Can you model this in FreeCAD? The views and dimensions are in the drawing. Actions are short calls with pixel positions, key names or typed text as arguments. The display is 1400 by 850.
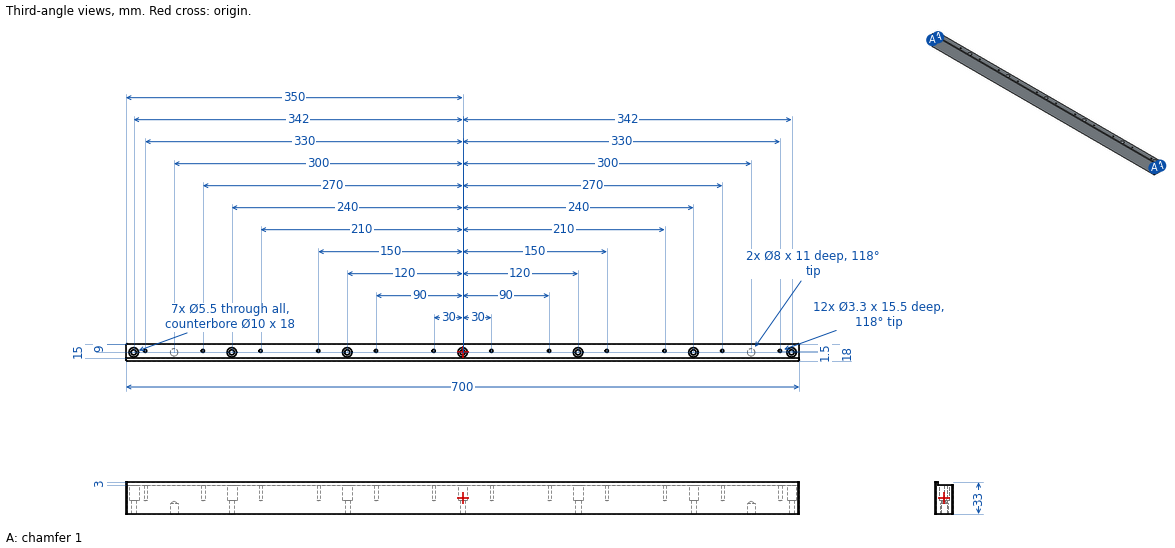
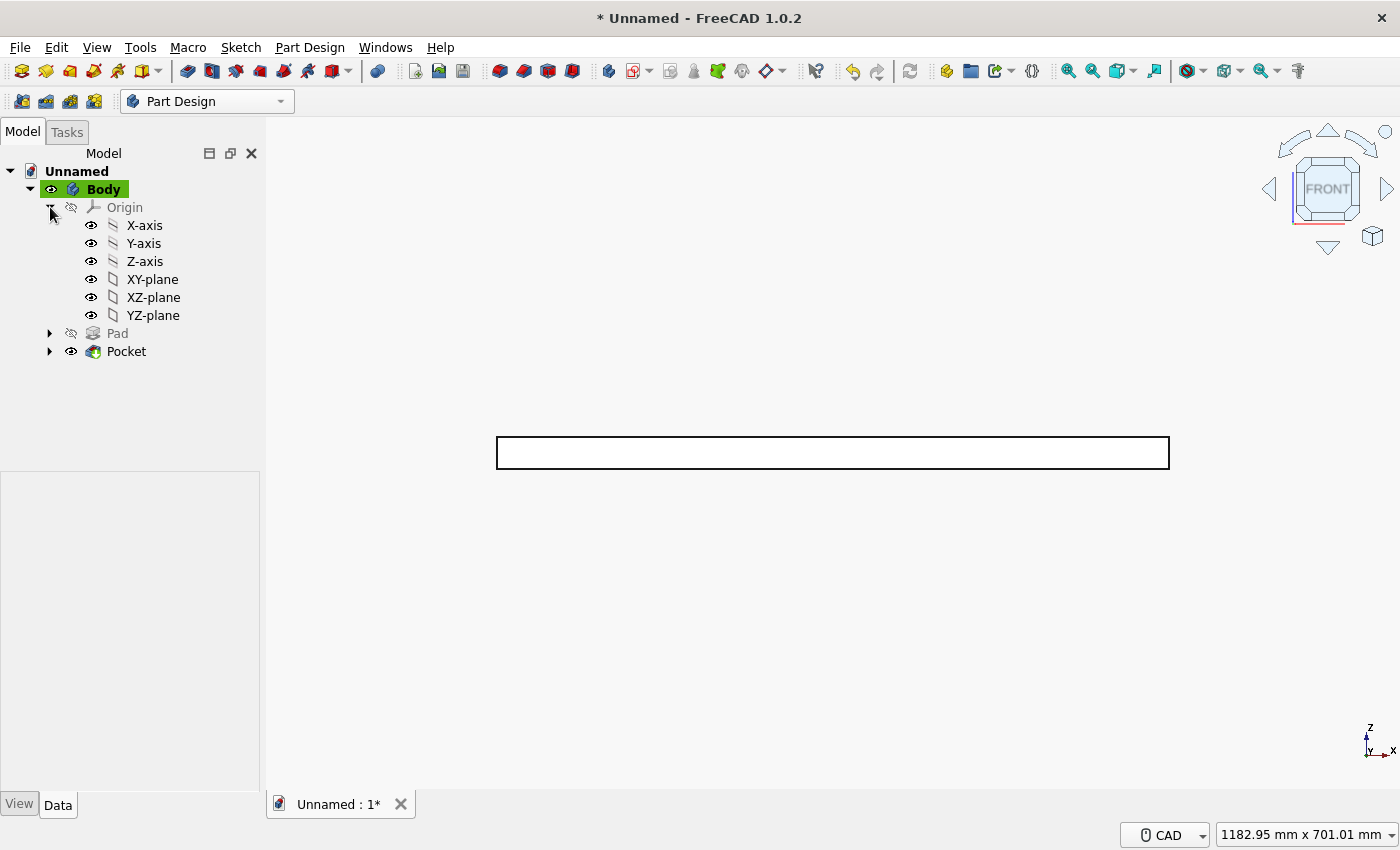
click(136, 279)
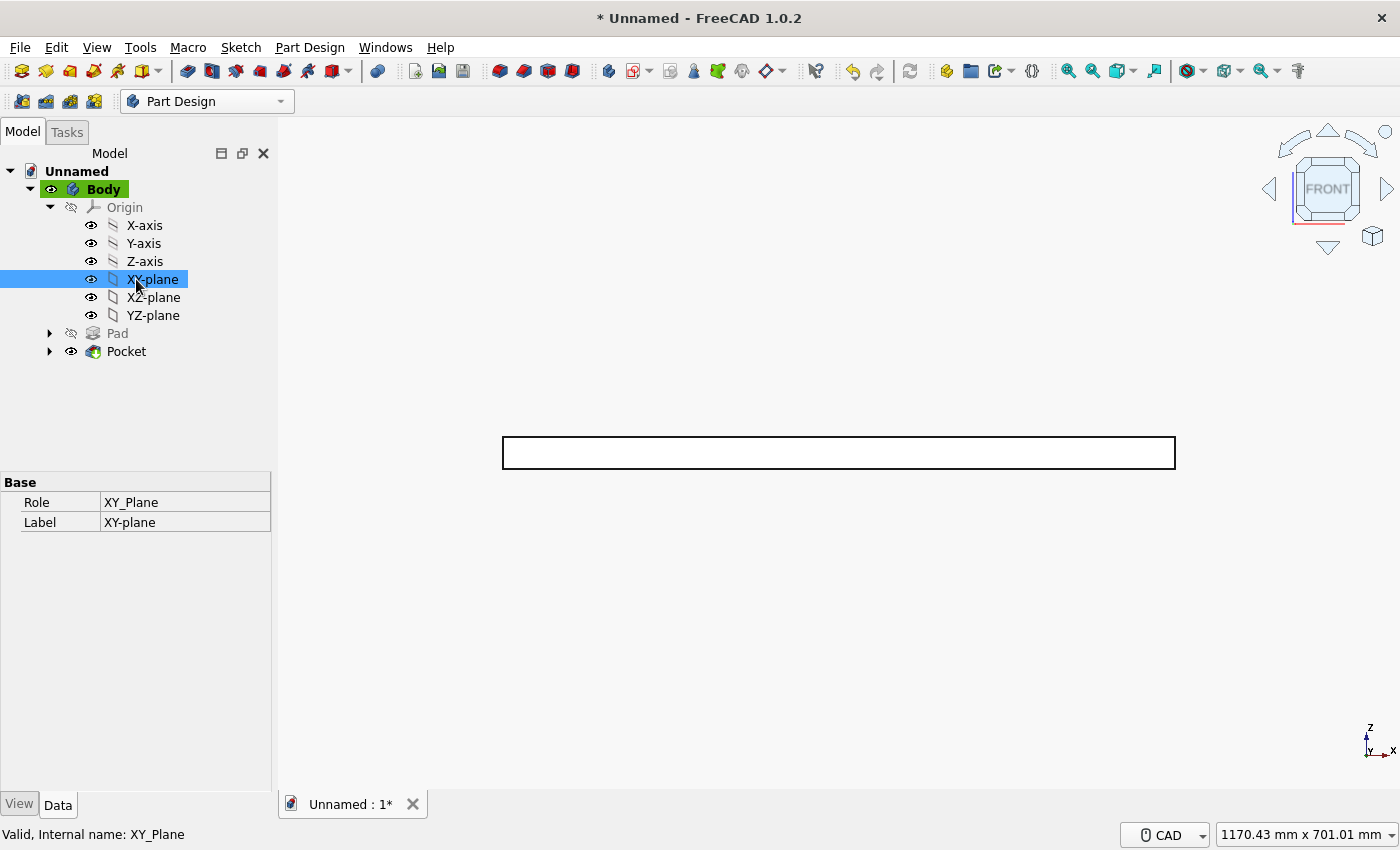
click(766, 72)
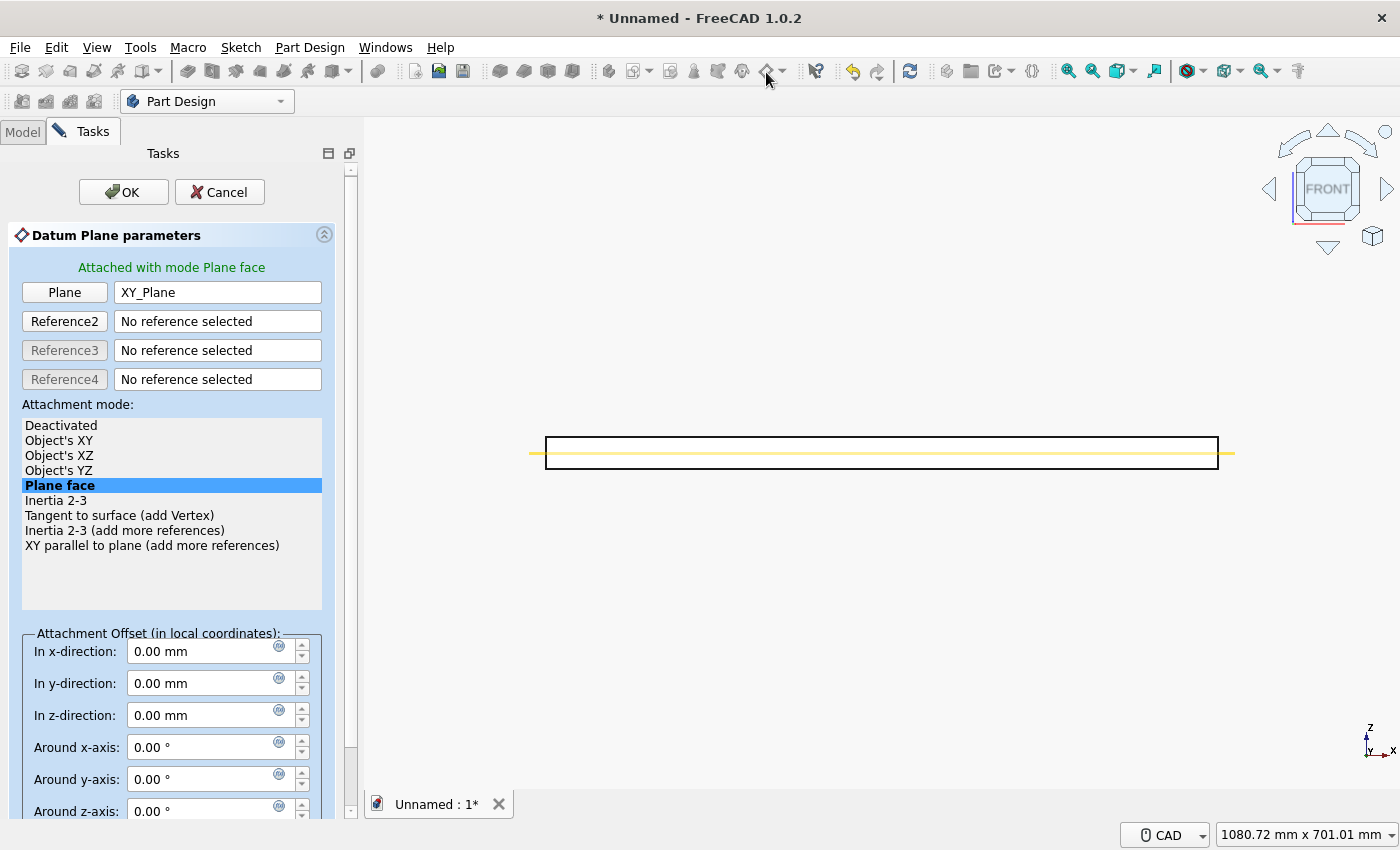
triple_click(210, 715)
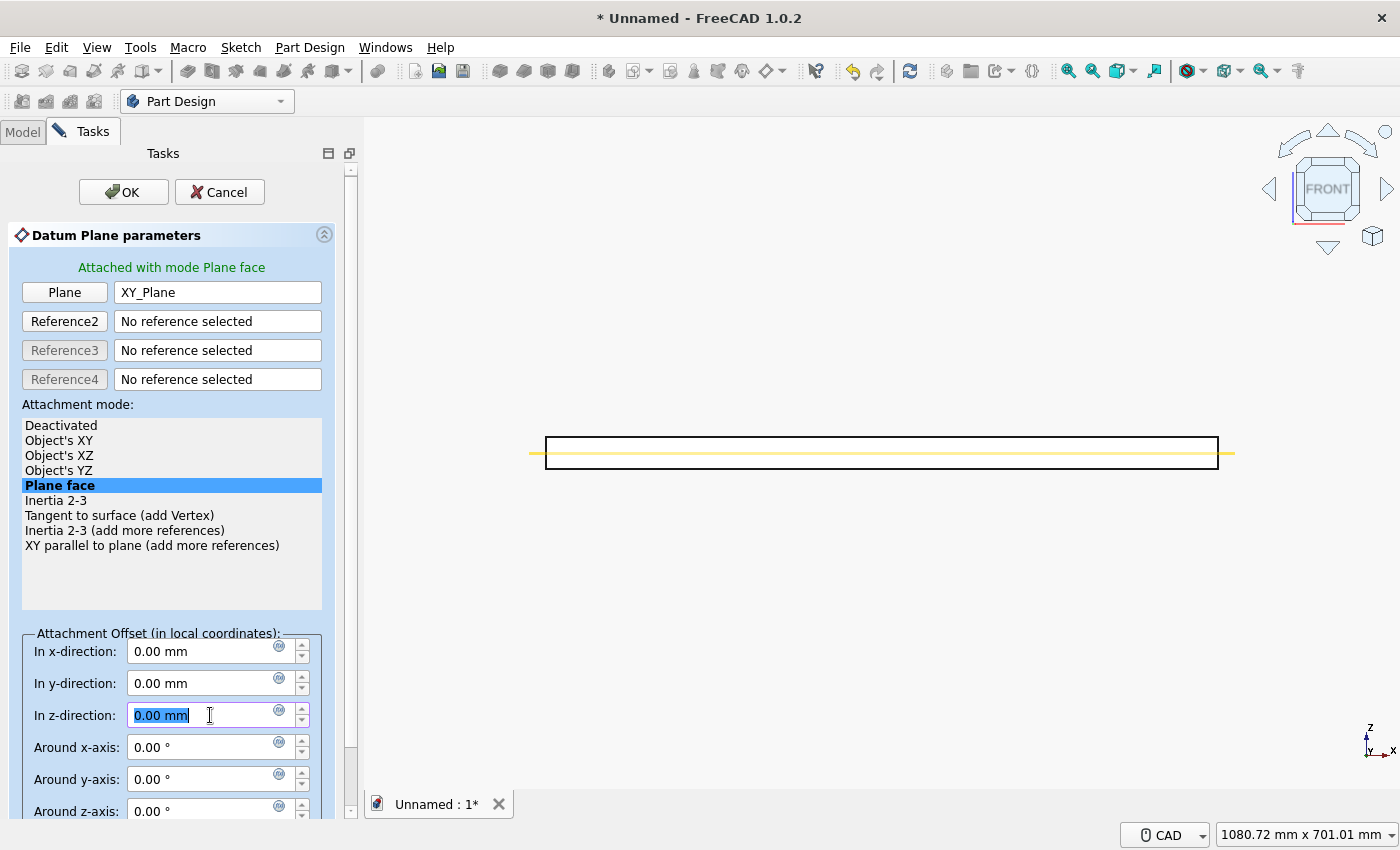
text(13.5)
key(Tab)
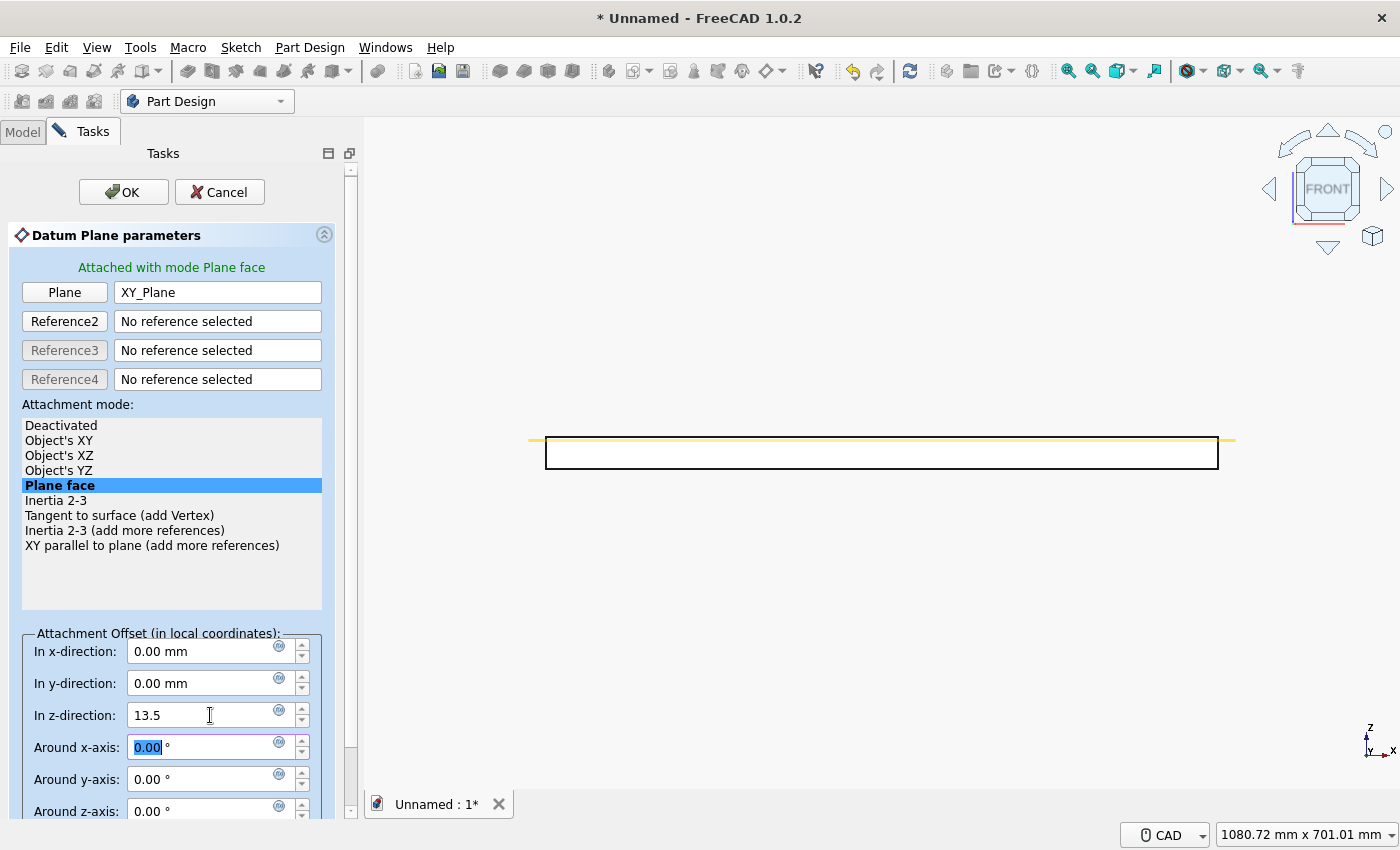
click(124, 192)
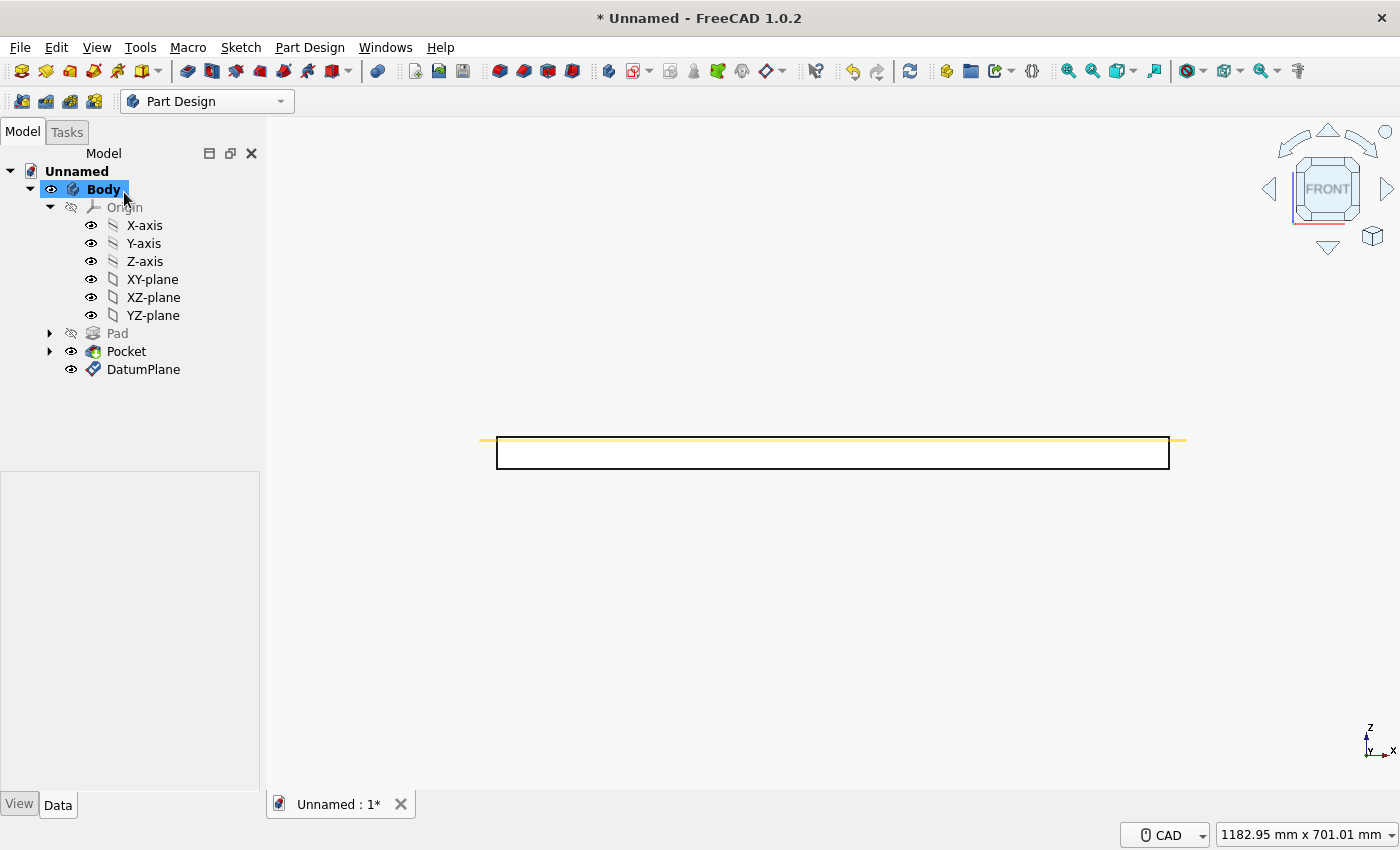
click(116, 369)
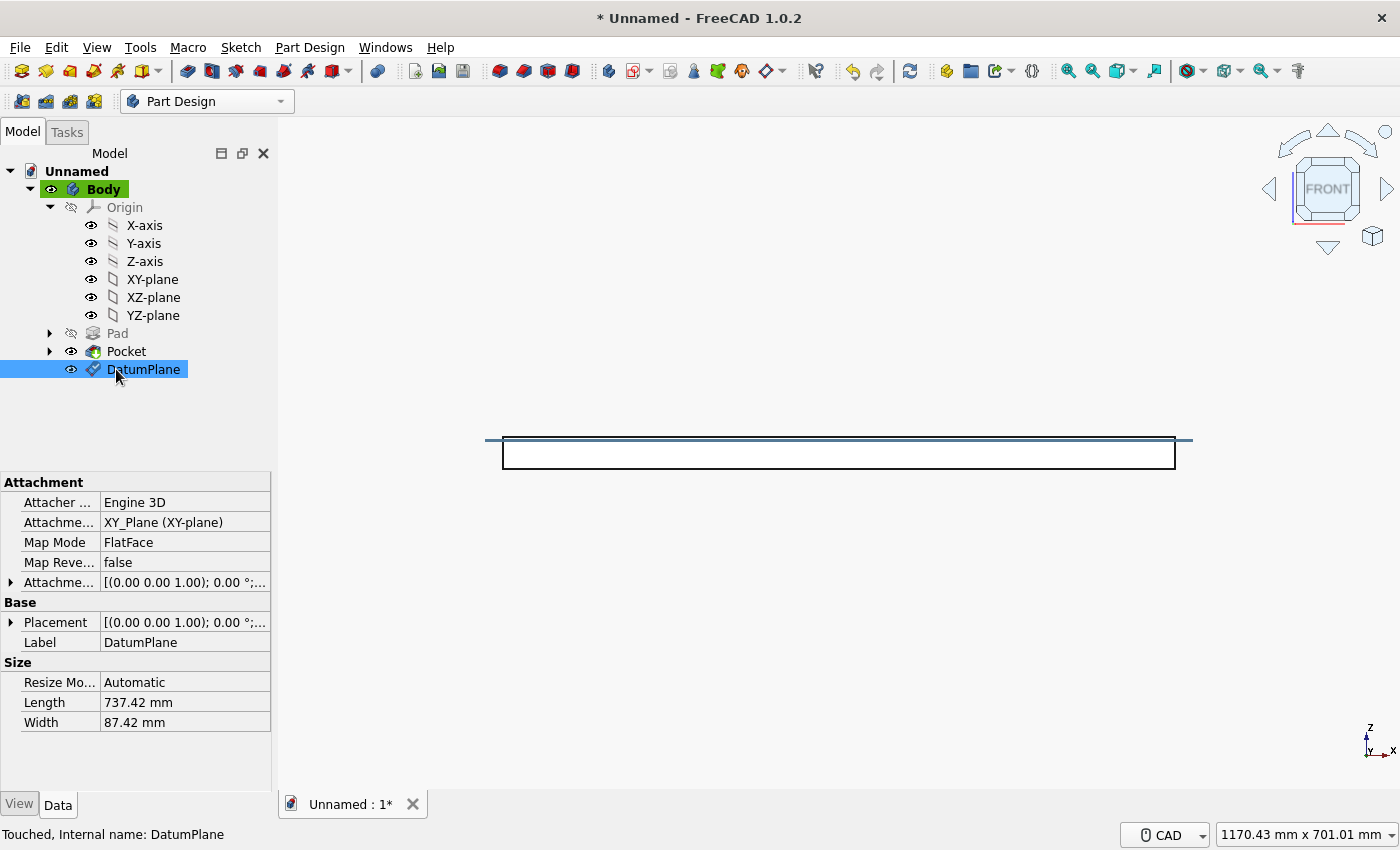
click(634, 72)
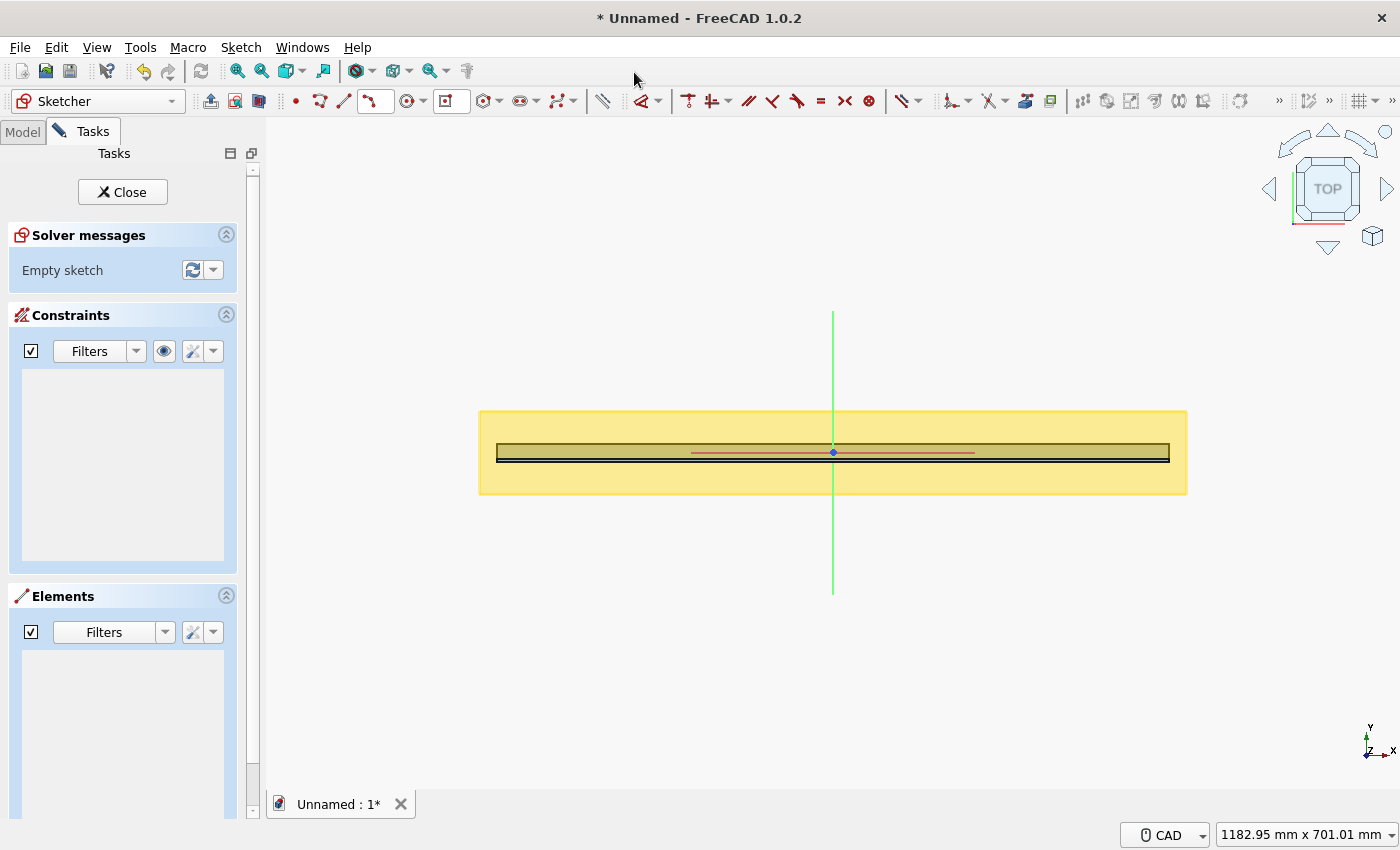
click(260, 102)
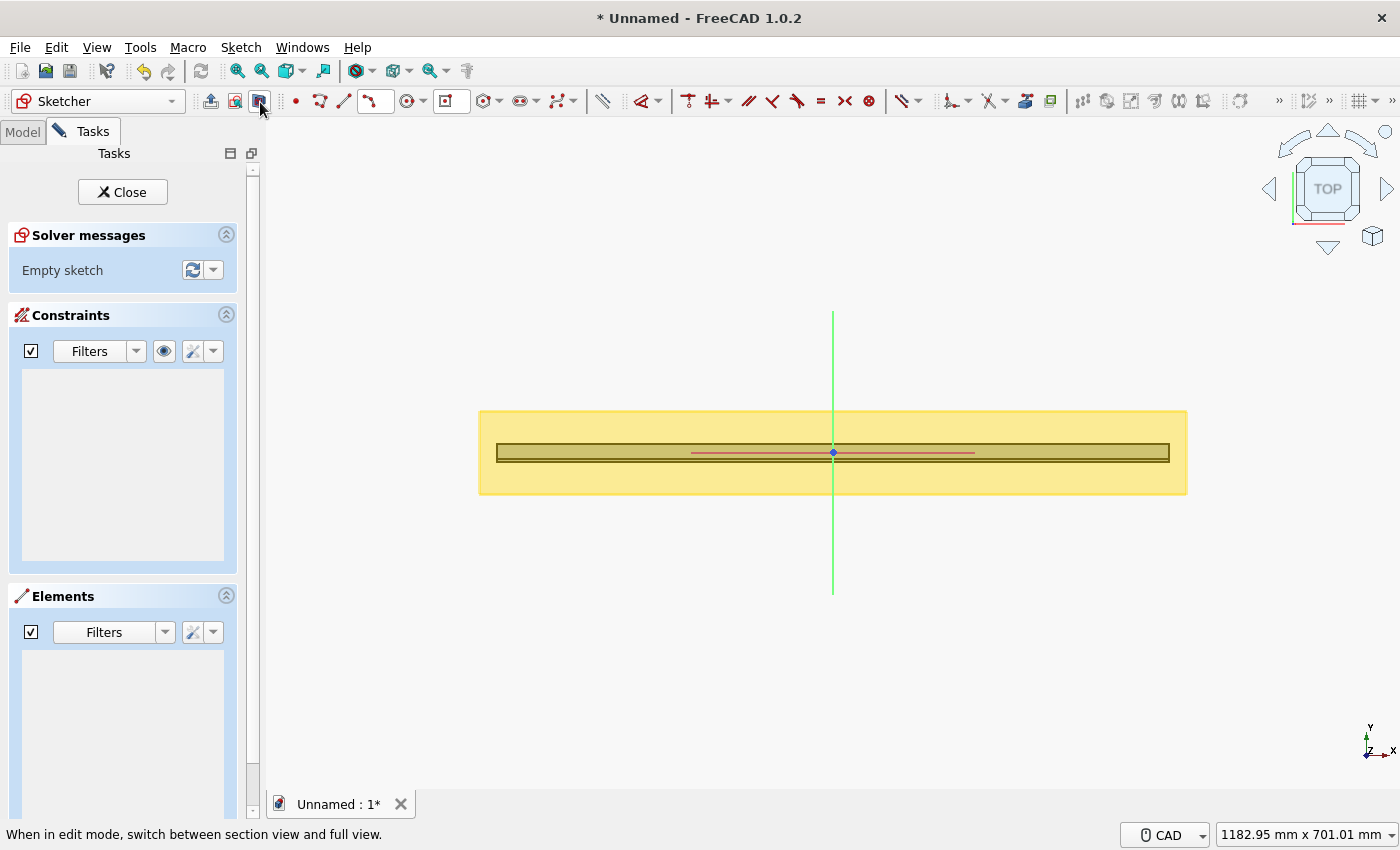
key(g)
key(c)